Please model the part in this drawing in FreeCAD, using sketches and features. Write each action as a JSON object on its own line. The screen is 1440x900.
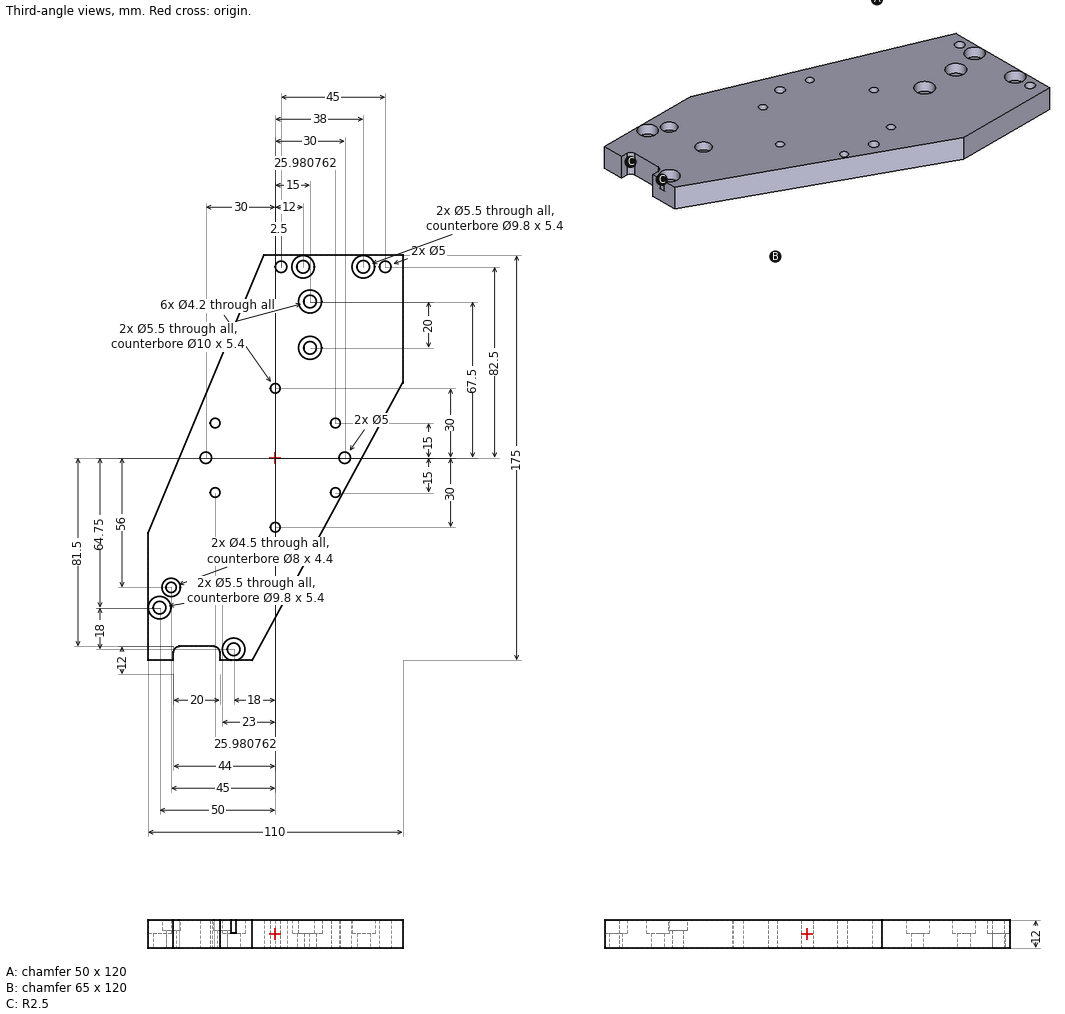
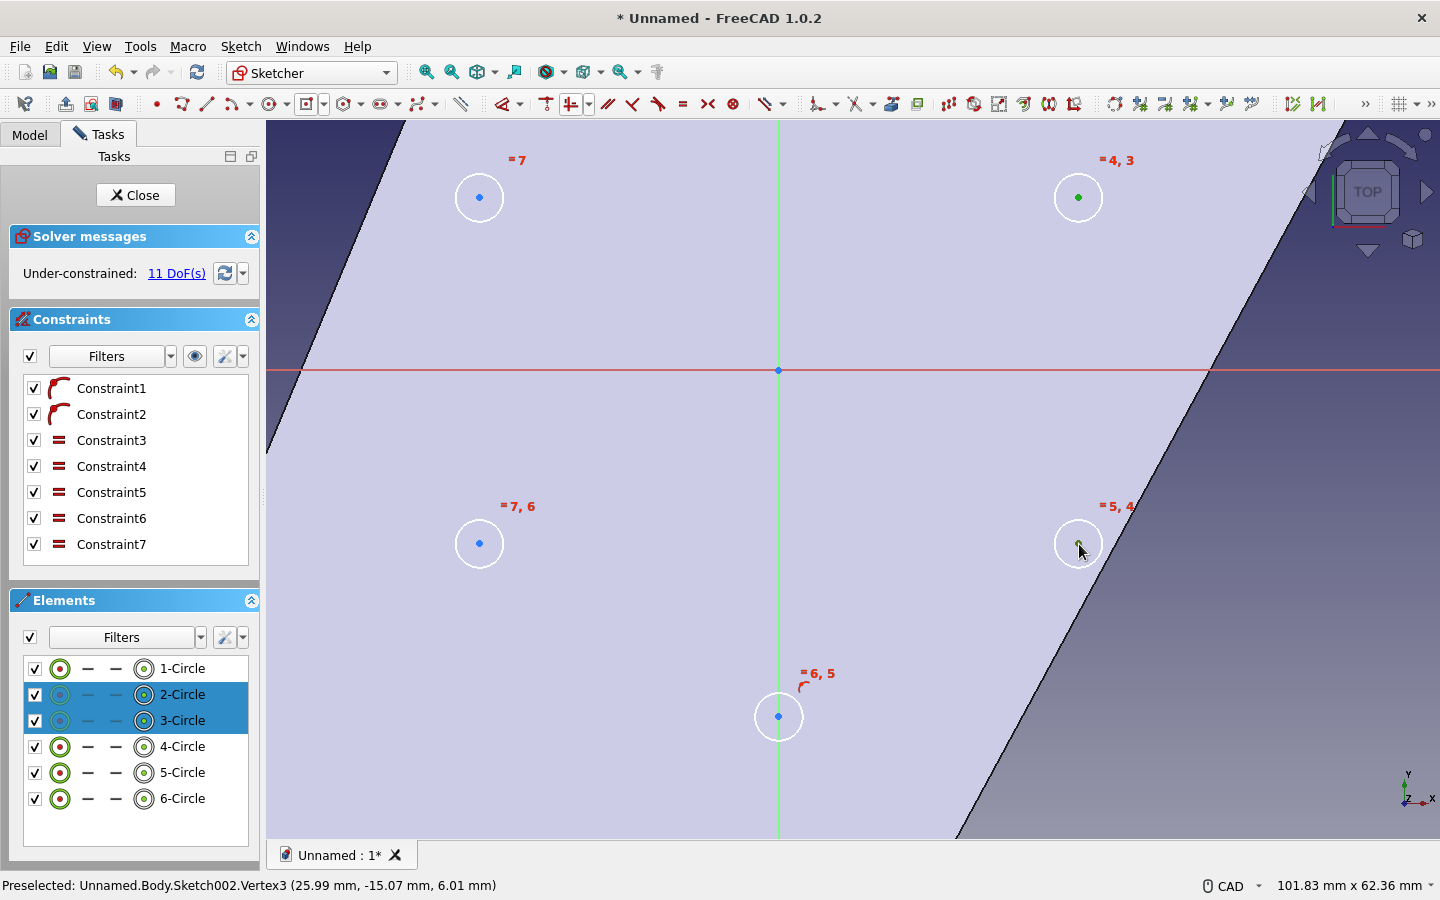
{"action": "key", "text": "v"}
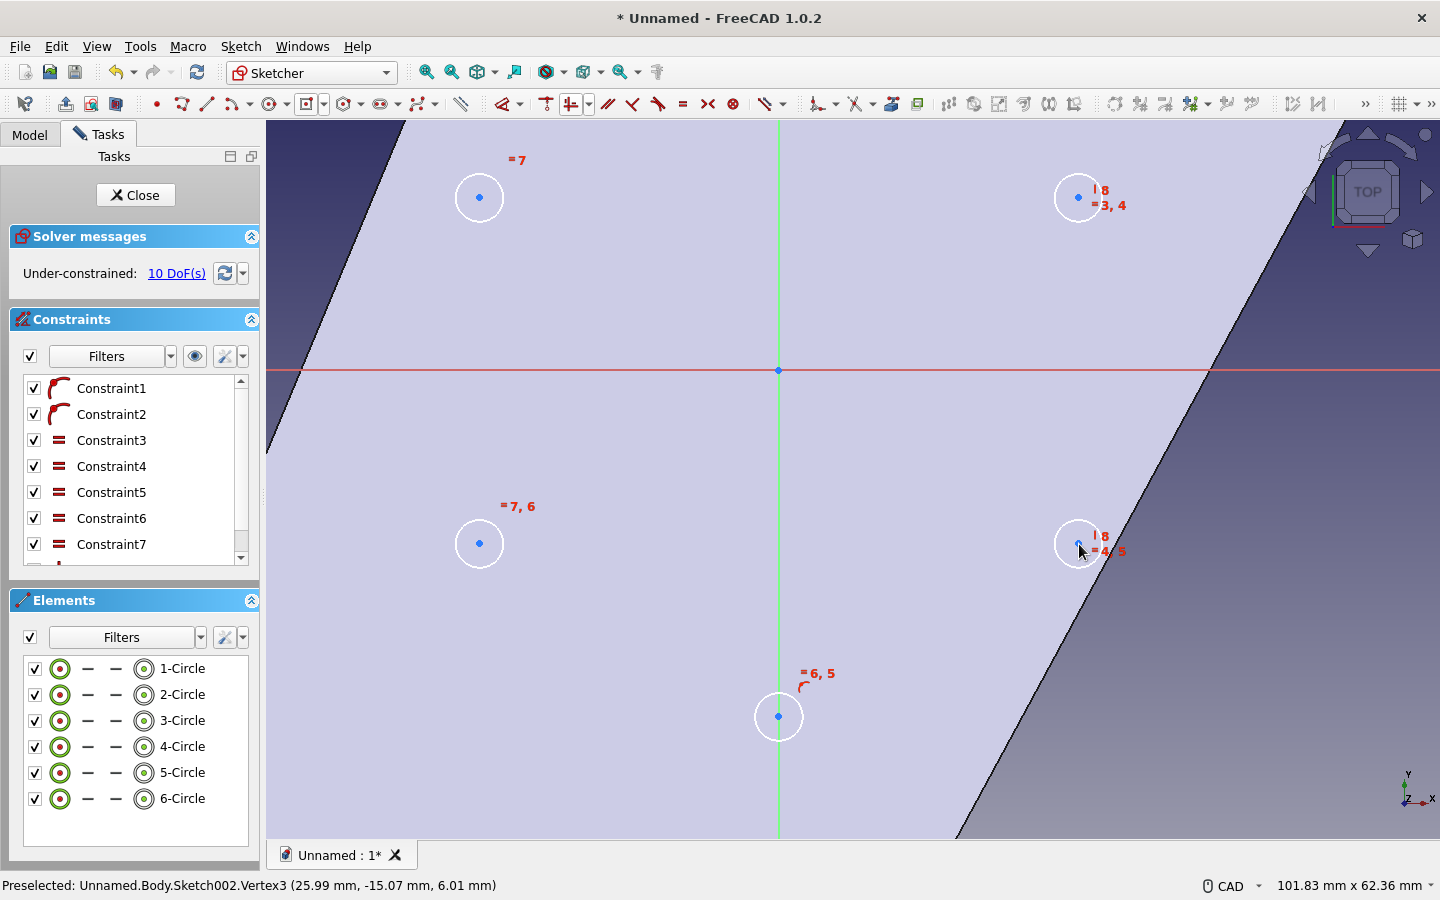
{"action": "left_click", "coordinate": [1079, 544]}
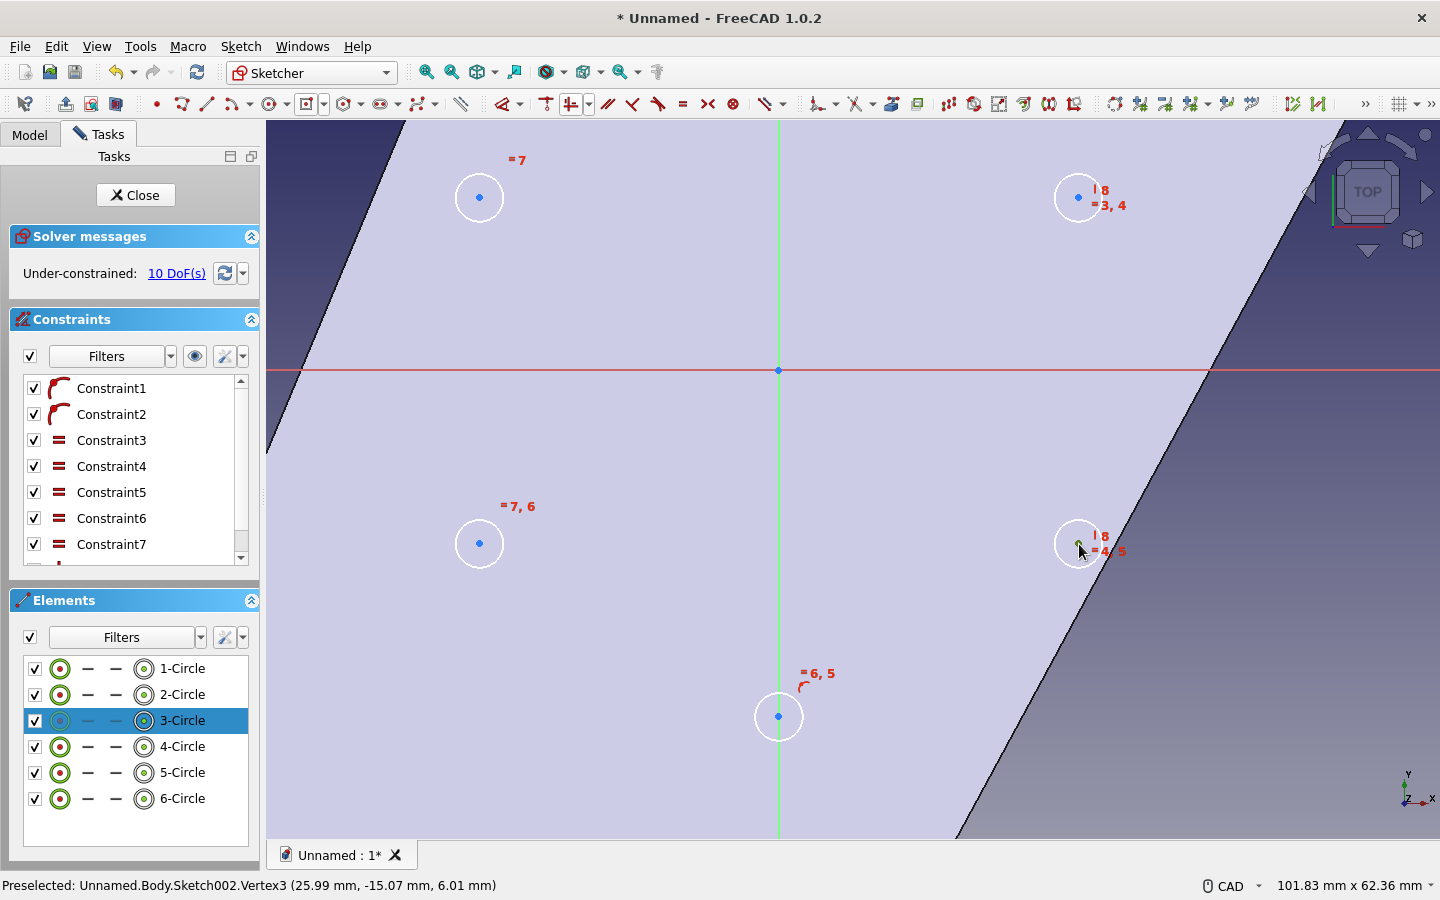
{"action": "left_click", "coordinate": [480, 544]}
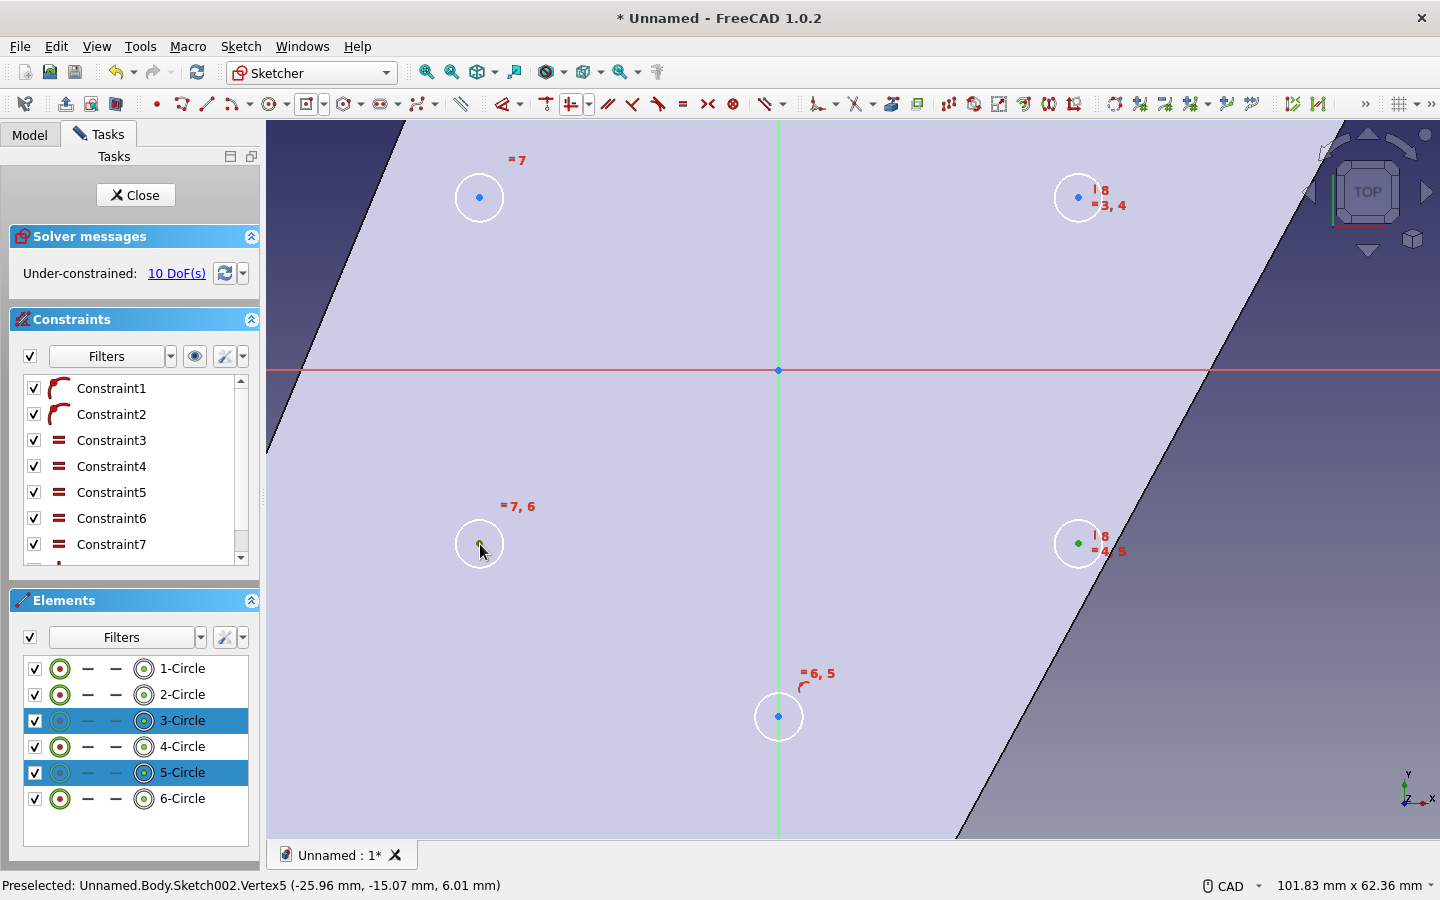
{"action": "key", "text": "h"}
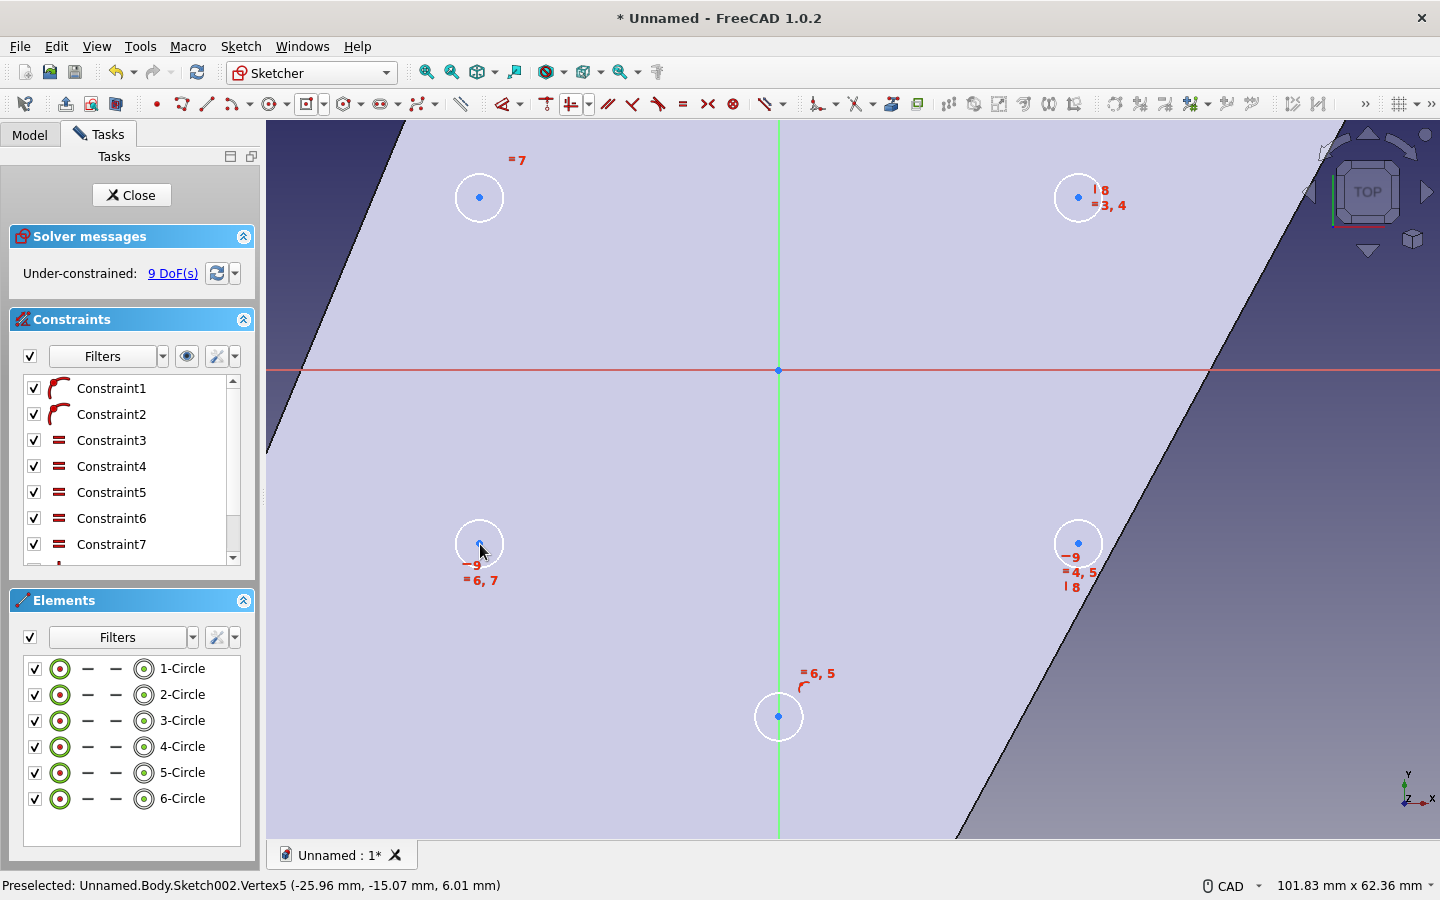
{"action": "left_click", "coordinate": [480, 544]}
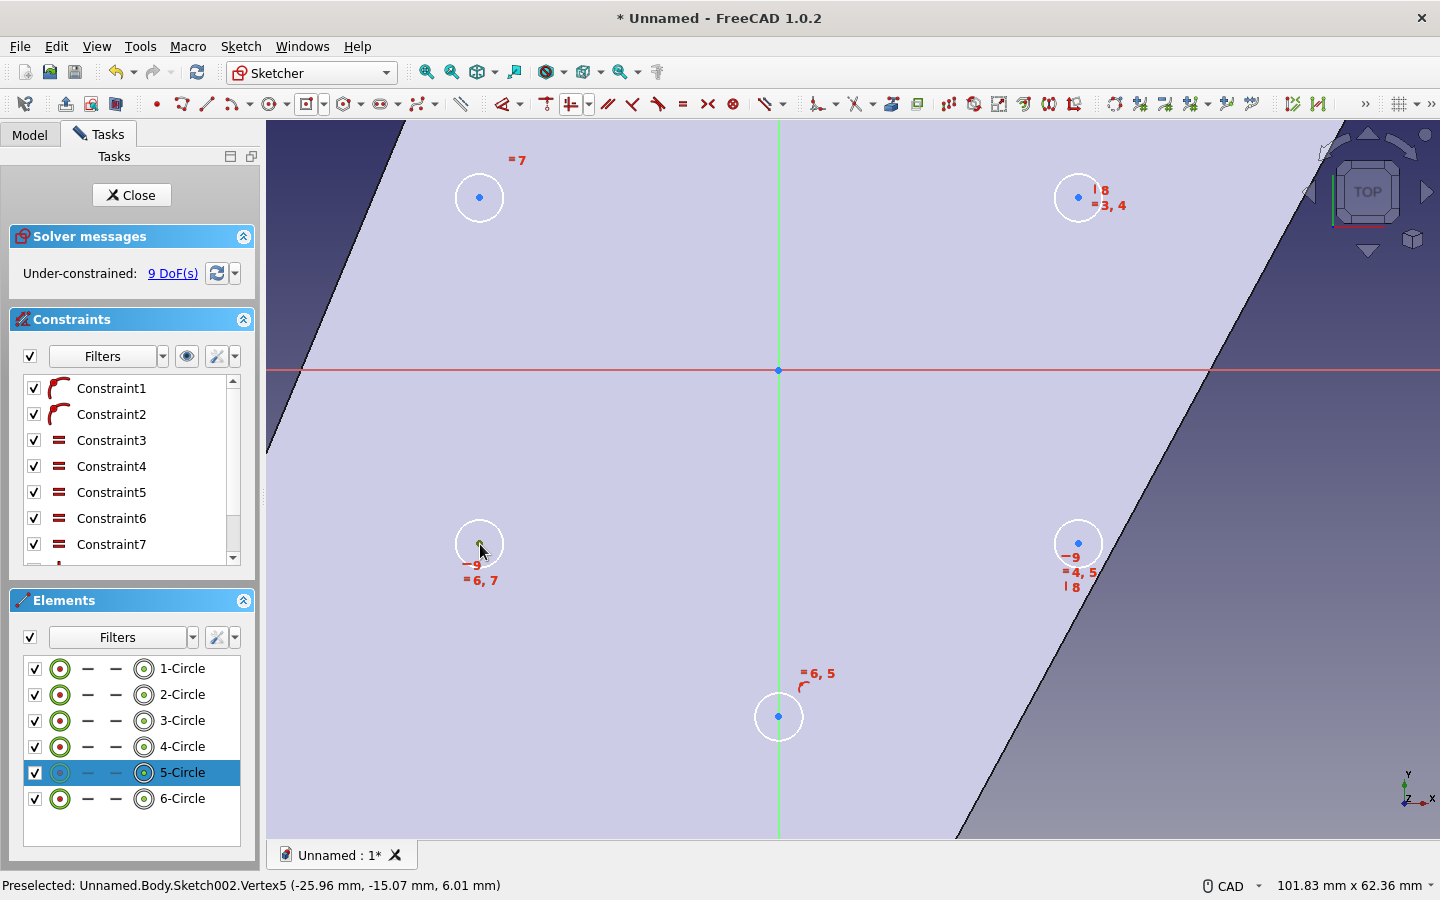
{"action": "left_click", "coordinate": [480, 198]}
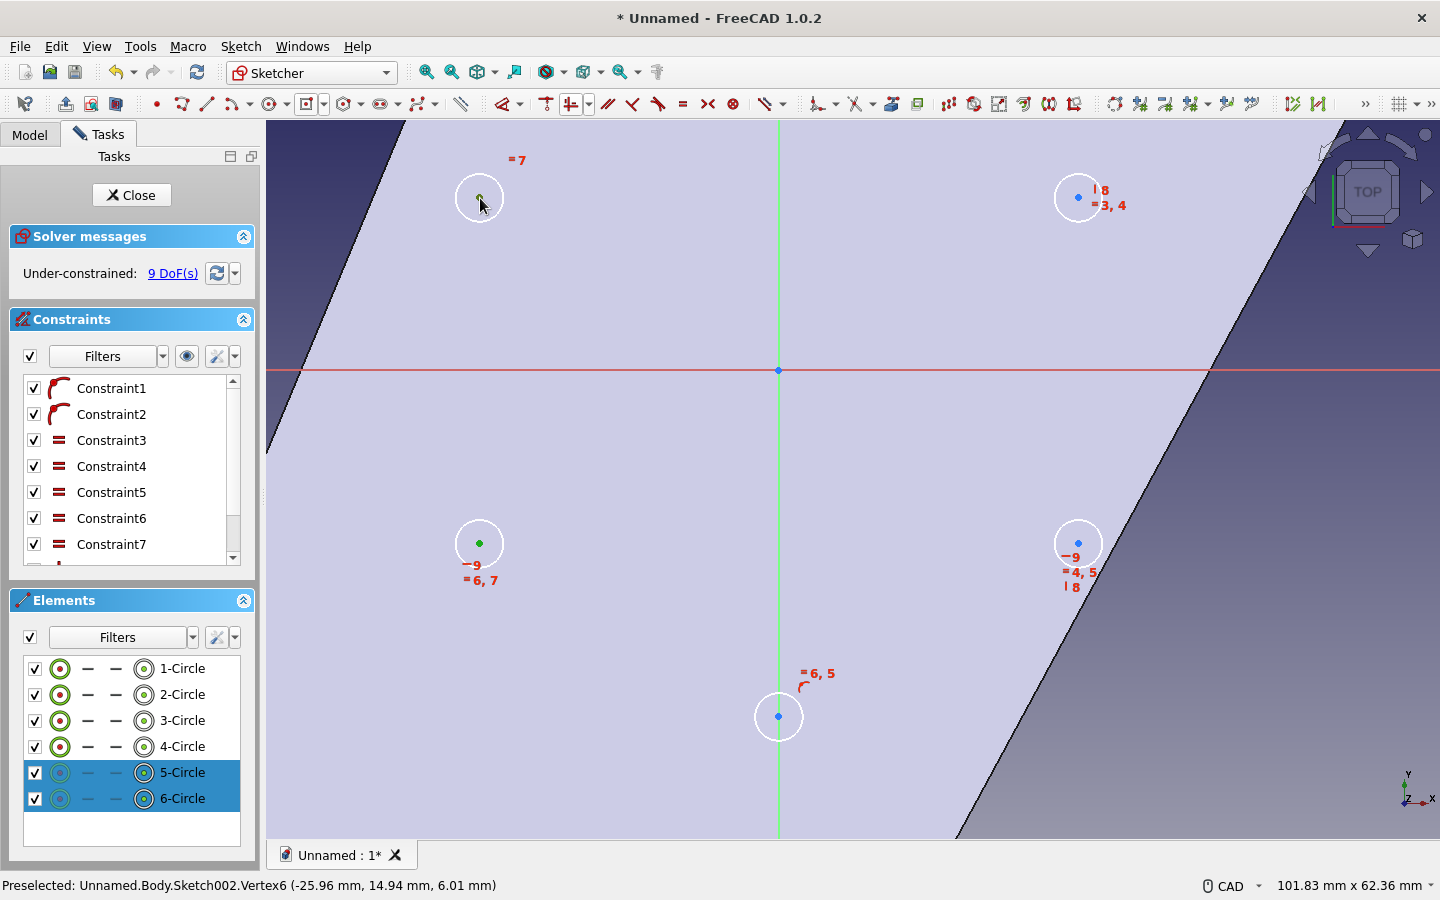
{"action": "key", "text": "v"}